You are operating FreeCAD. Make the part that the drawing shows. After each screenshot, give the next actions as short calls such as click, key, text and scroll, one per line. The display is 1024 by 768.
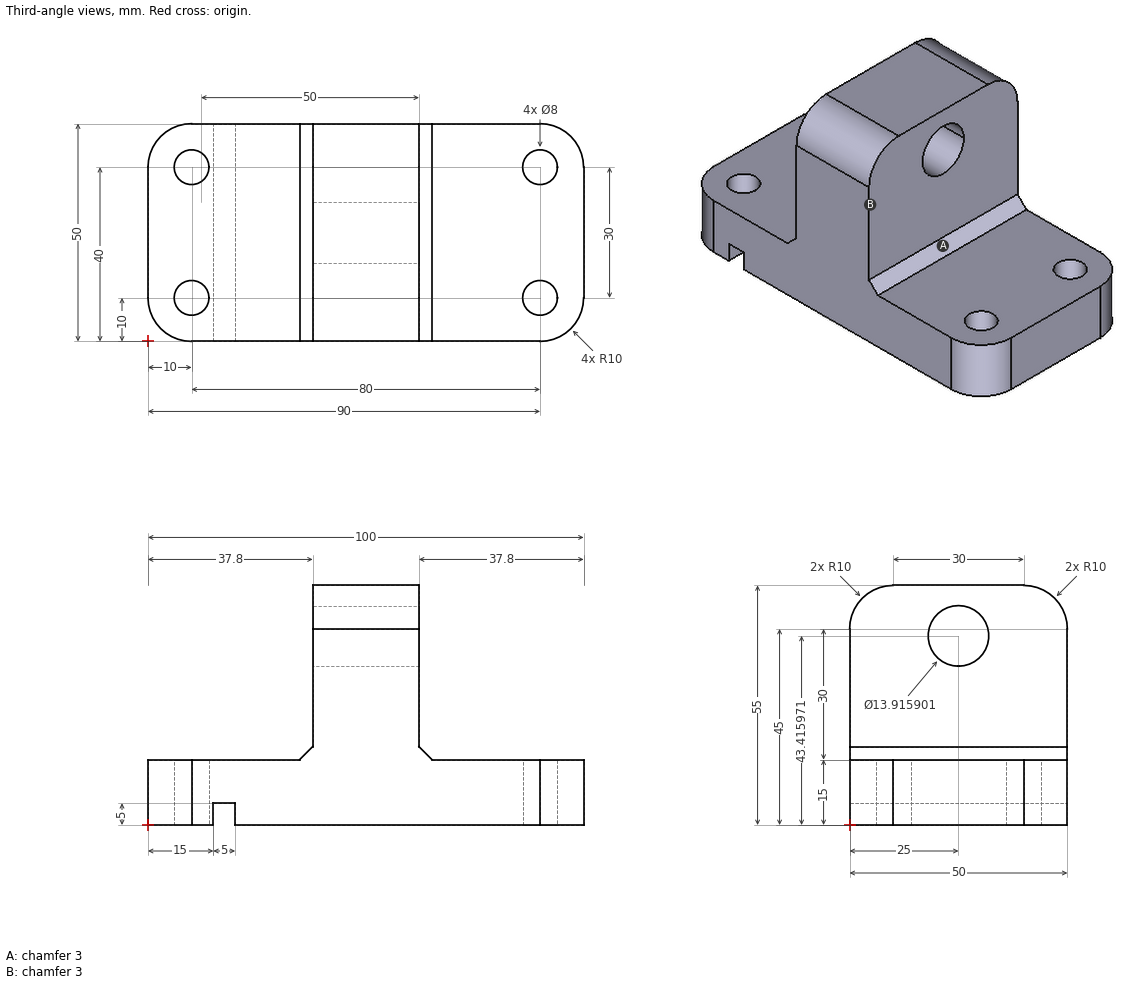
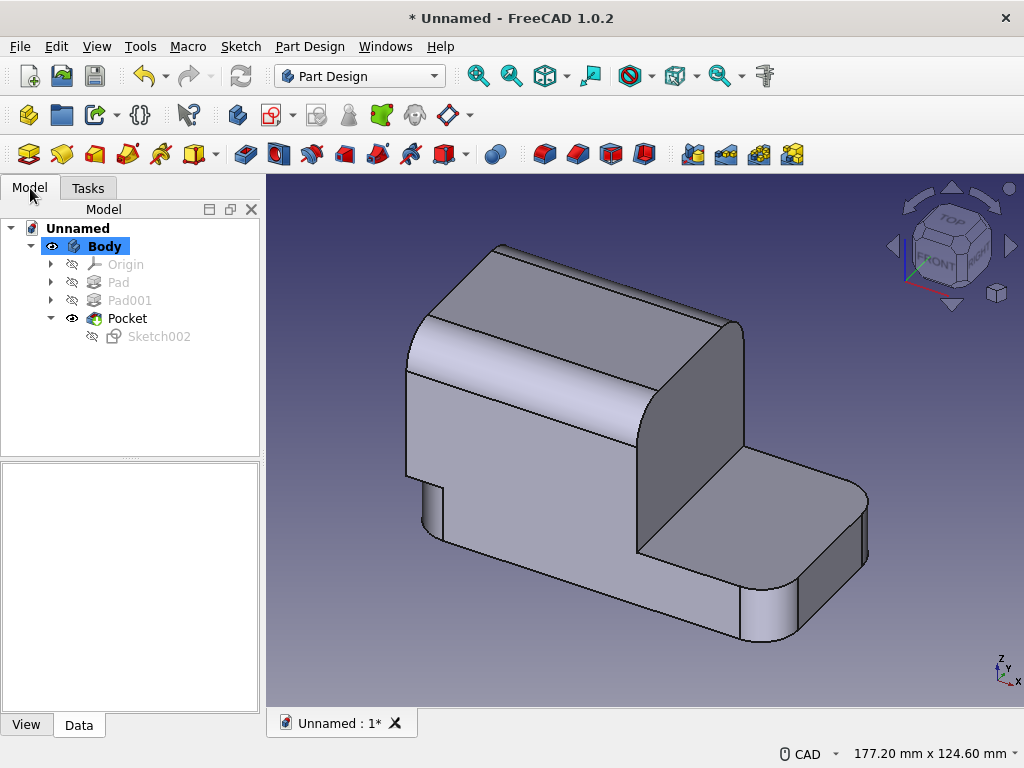
click(51, 264)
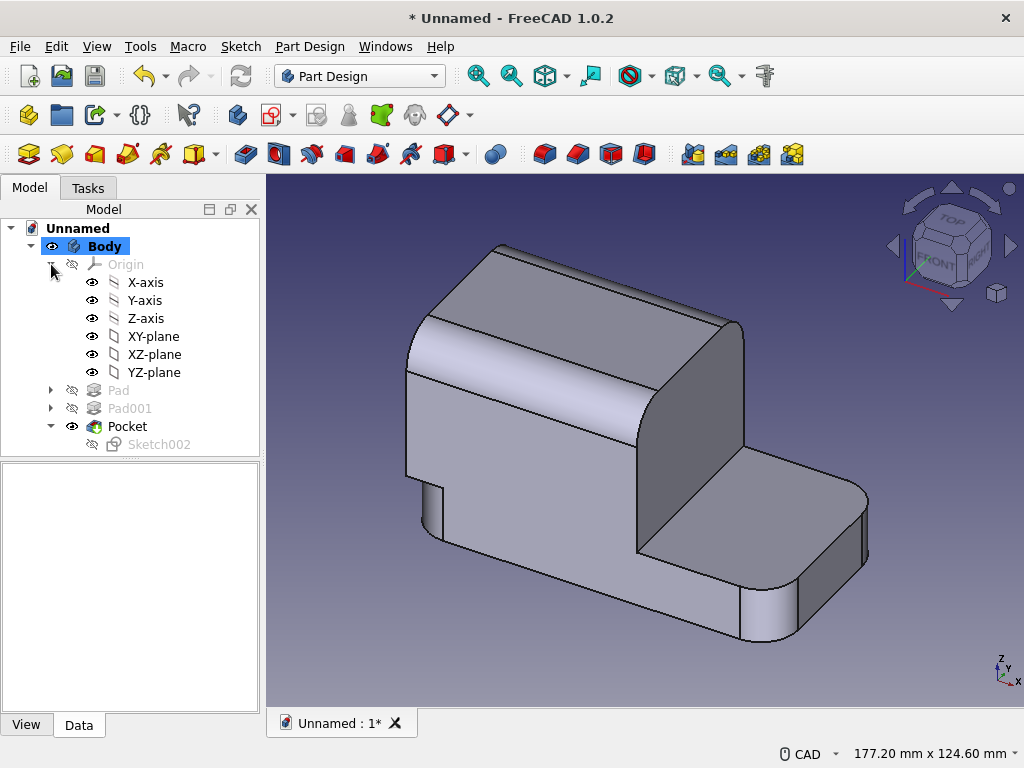
click(137, 372)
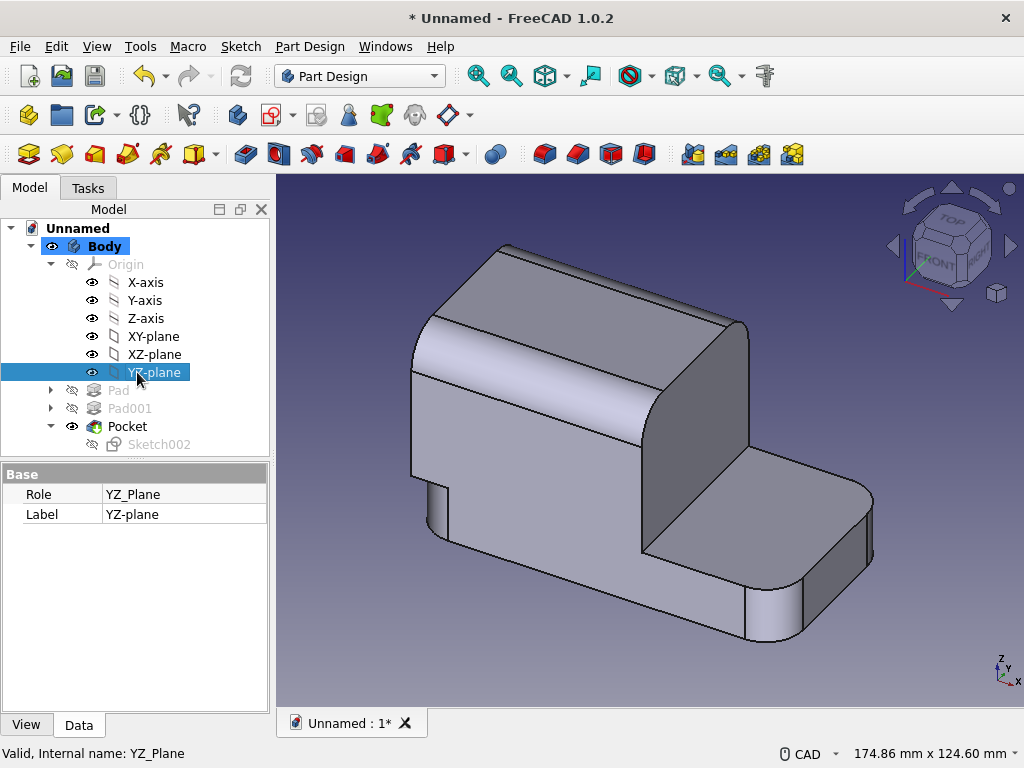
click(448, 116)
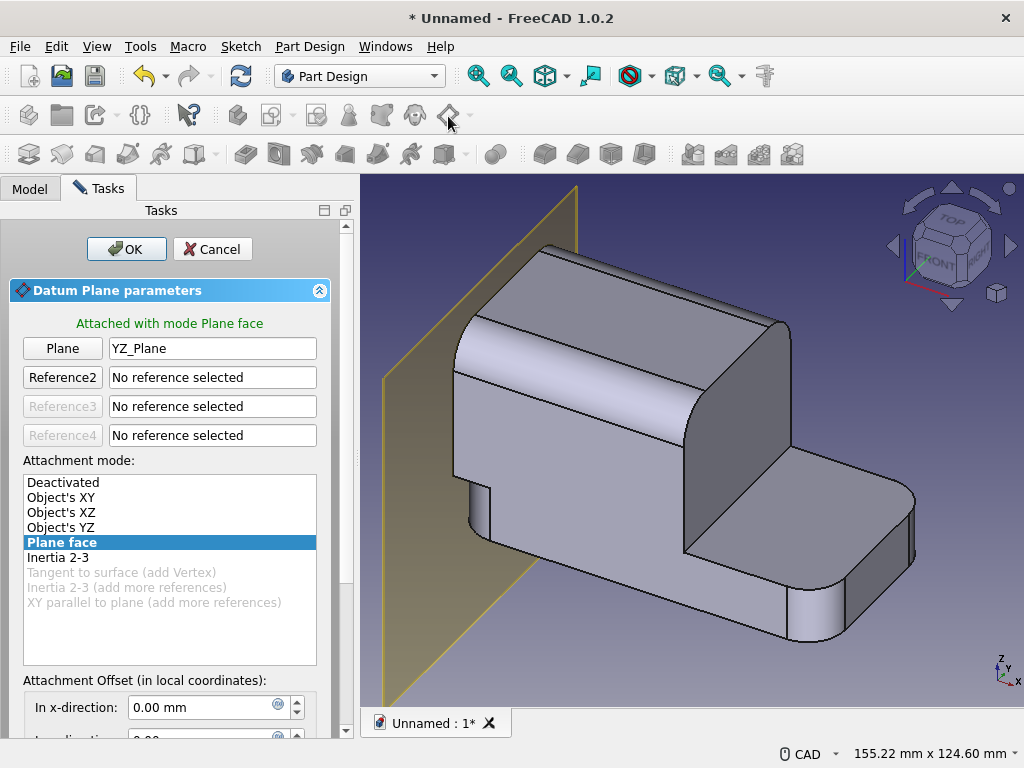
scroll(346, 479, down, 2)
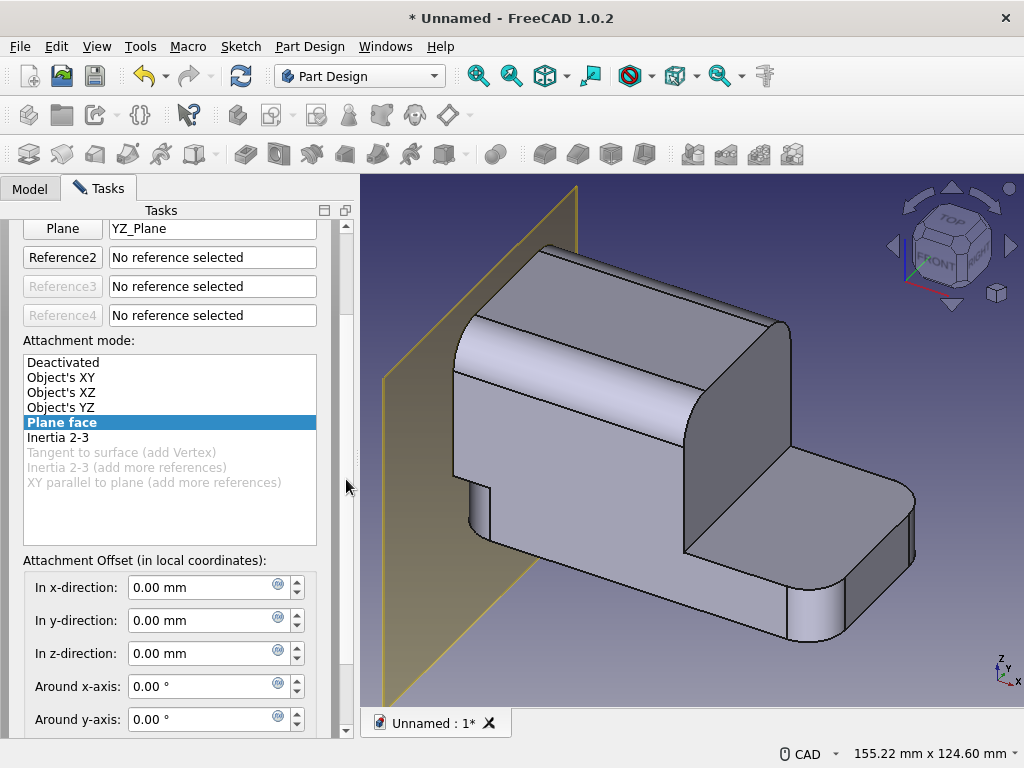
triple_click(210, 654)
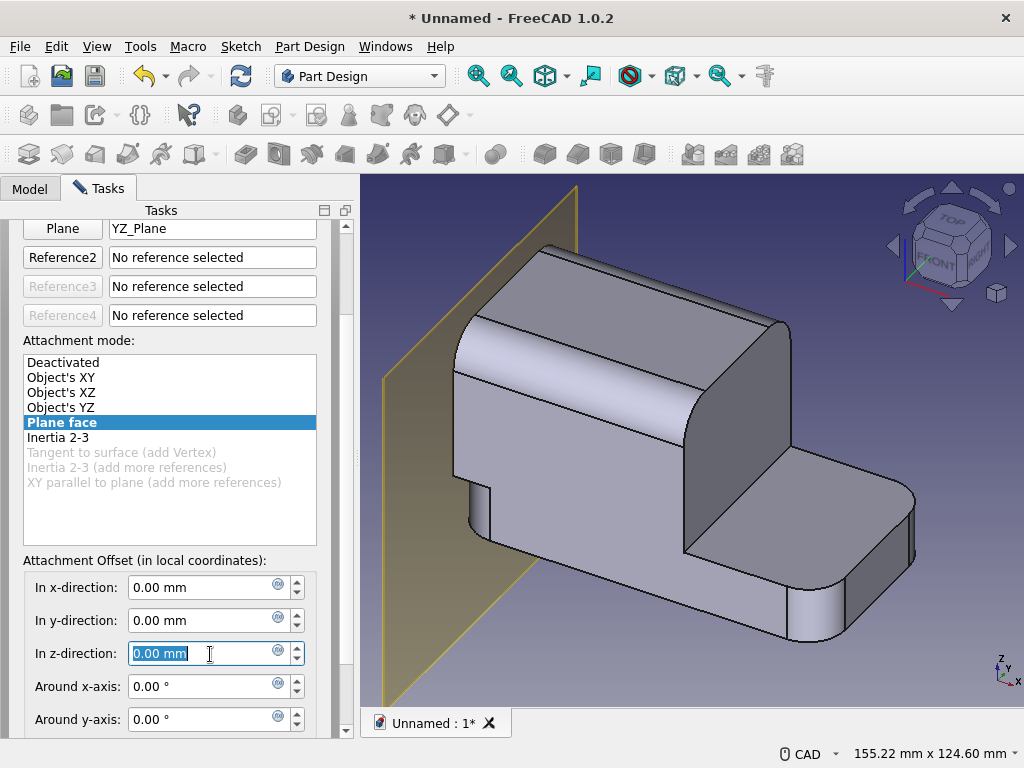
text(37.8)
key(Tab)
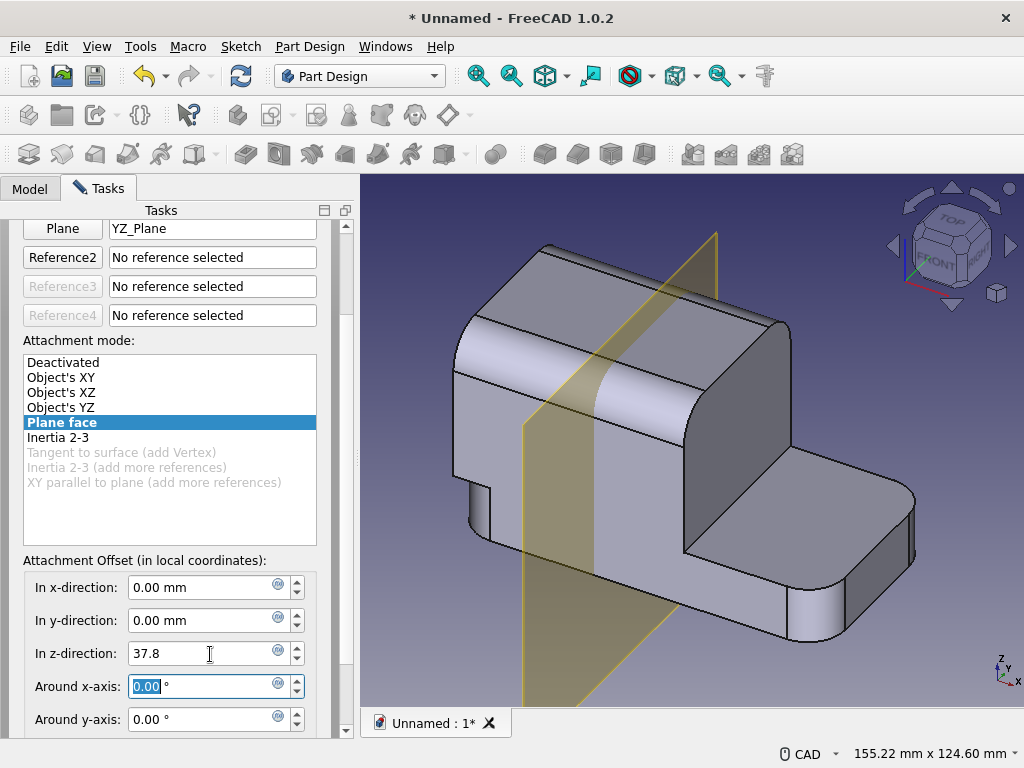
scroll(346, 479, up, 3)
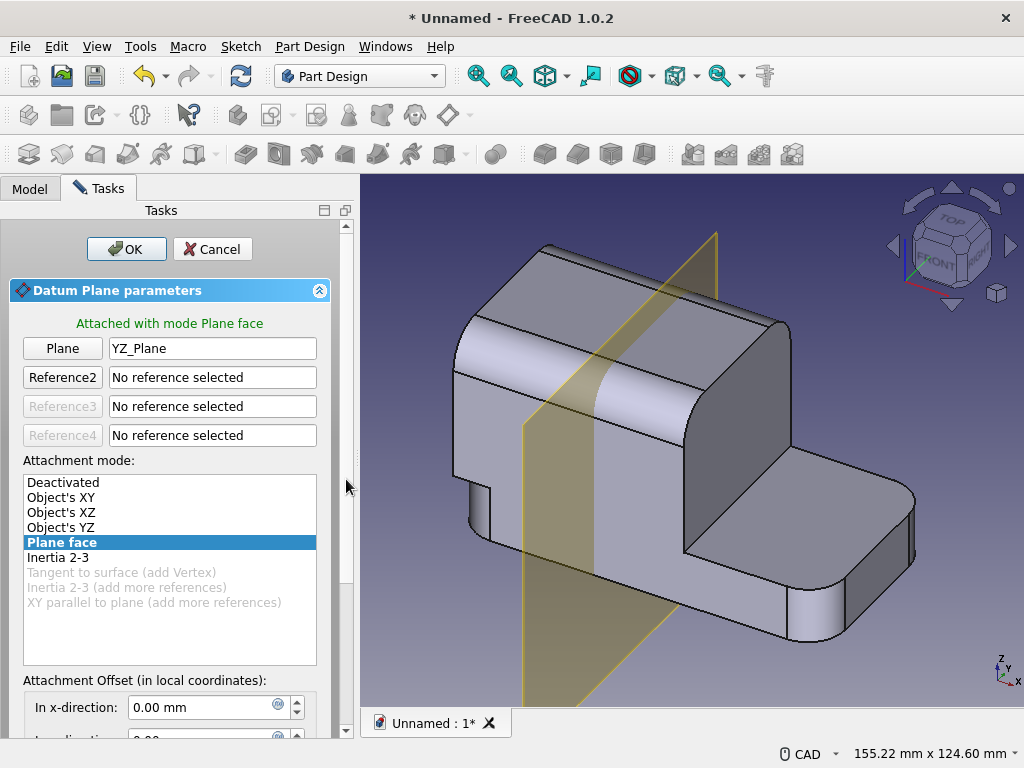
click(127, 249)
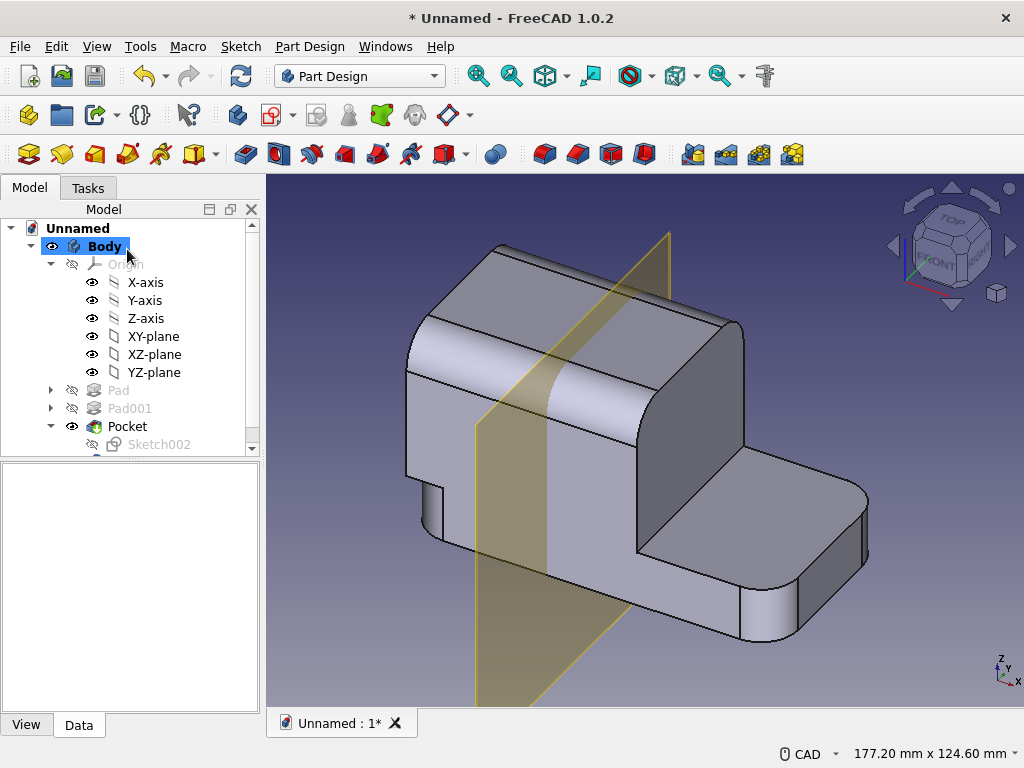
scroll(101, 332, down, 3)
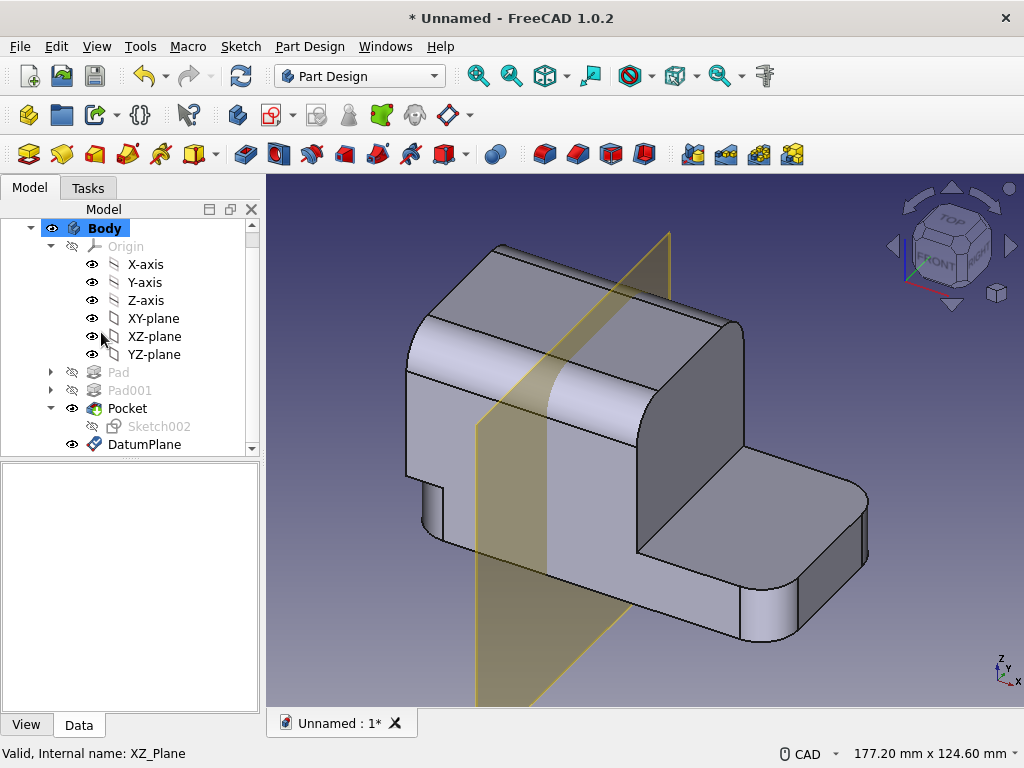
click(117, 444)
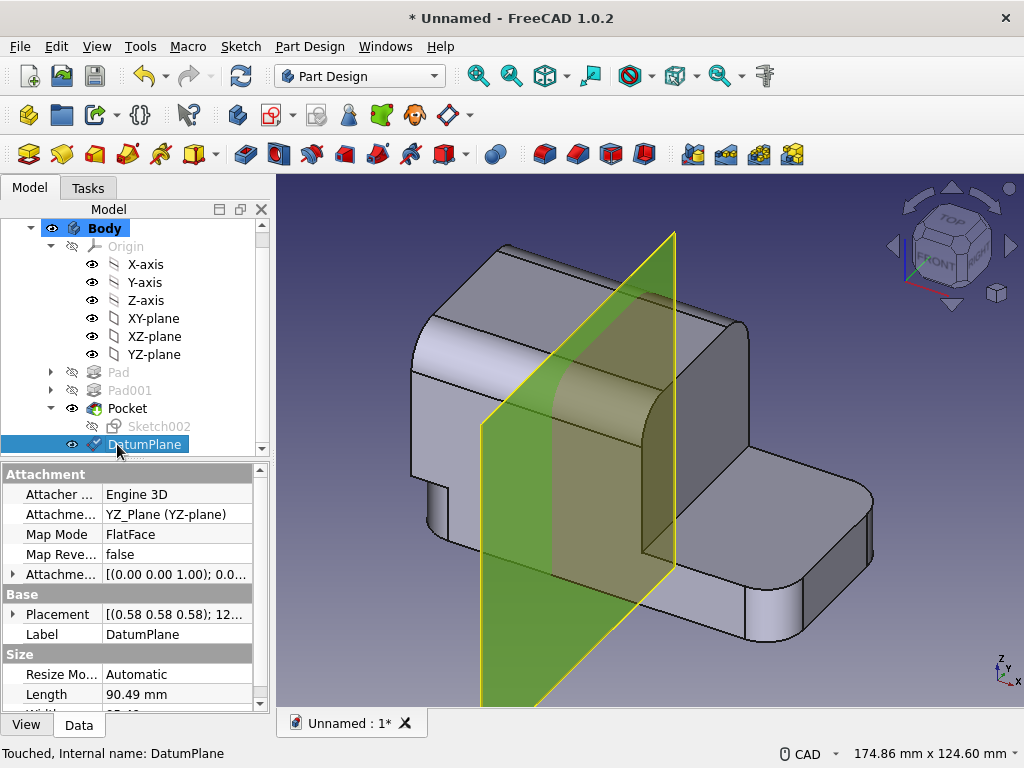
click(270, 116)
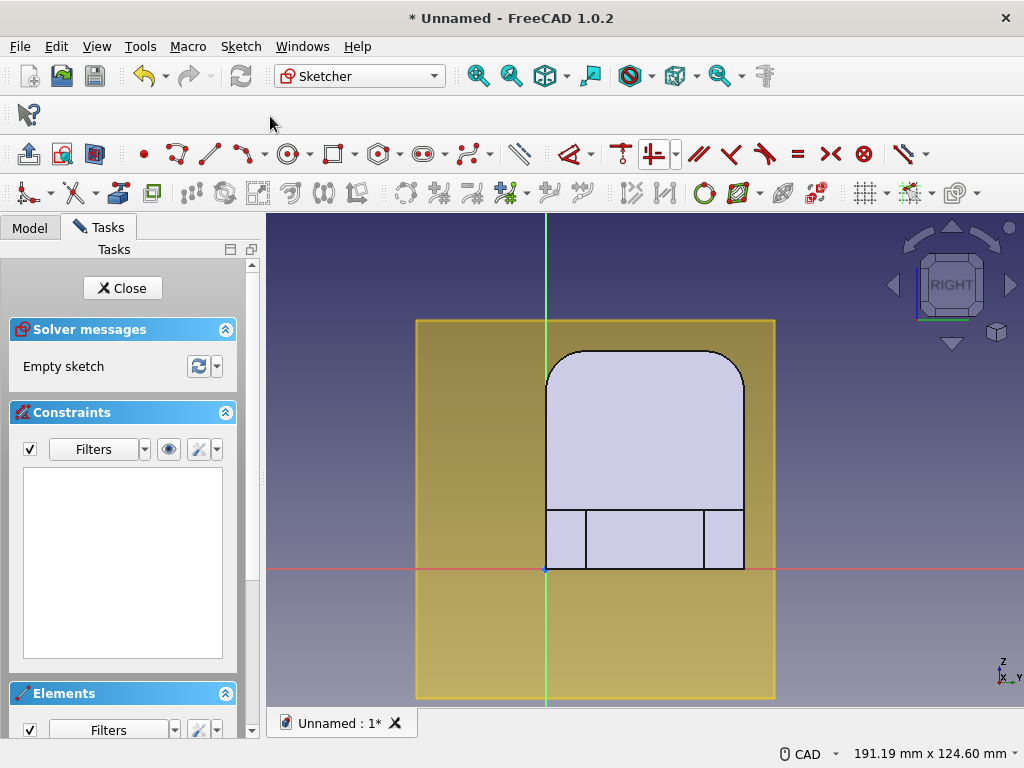
click(95, 154)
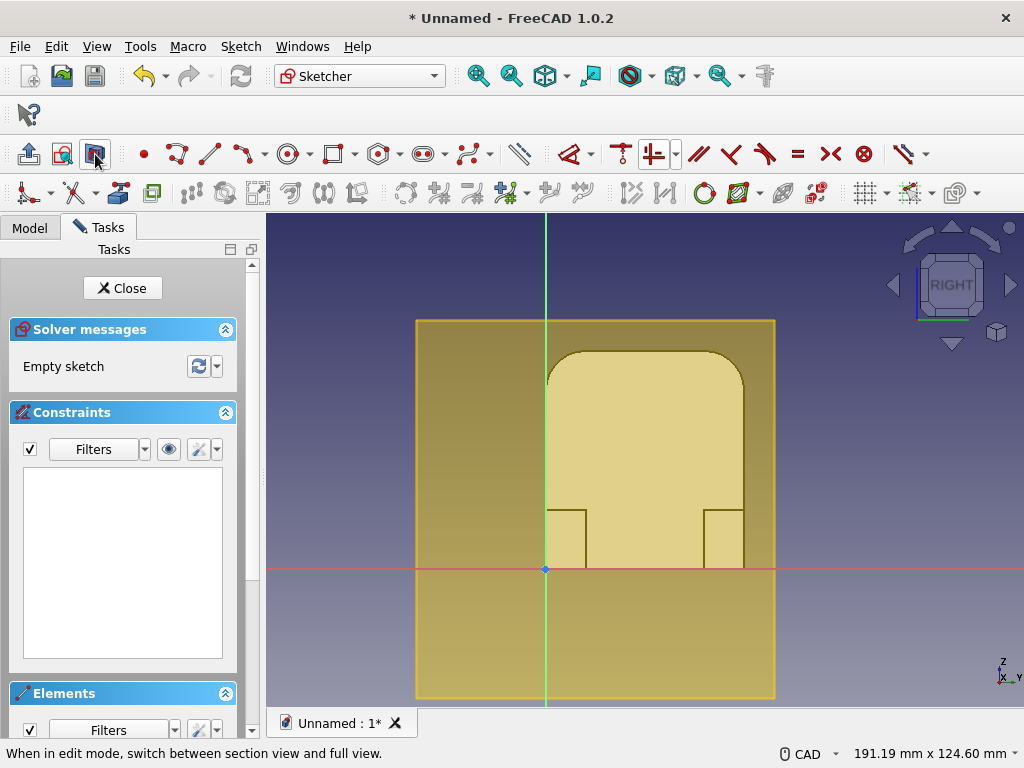
scroll(784, 460, up, 2)